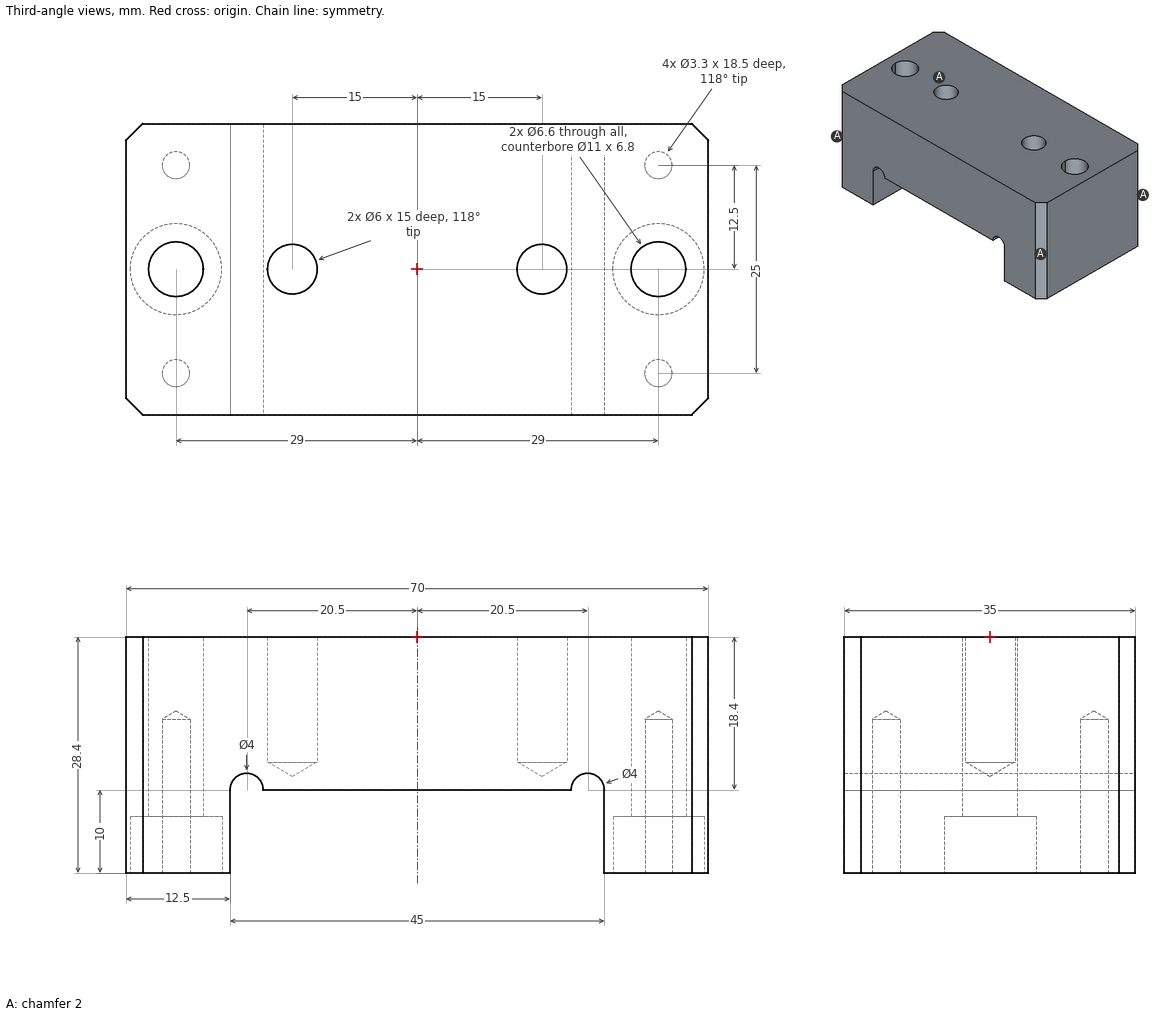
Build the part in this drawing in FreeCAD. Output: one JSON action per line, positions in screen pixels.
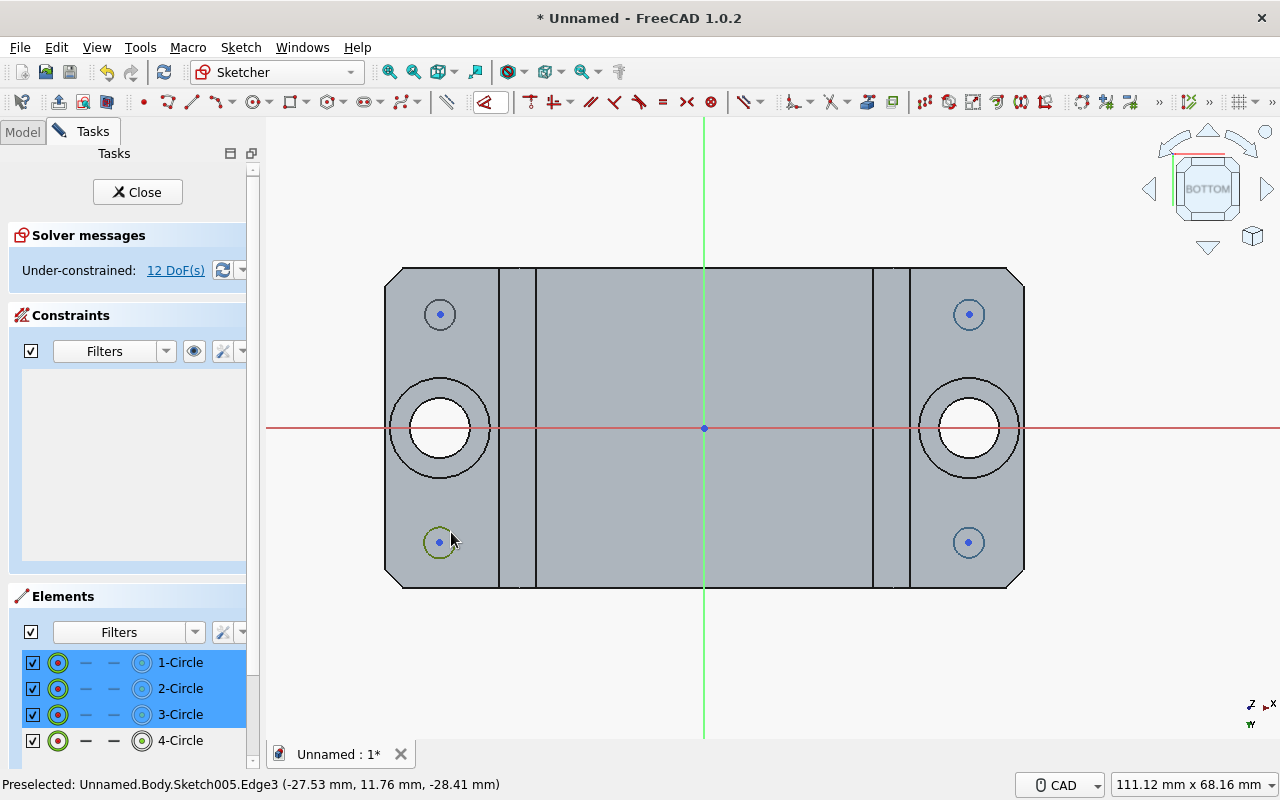
{"action": "left_click", "coordinate": [451, 304]}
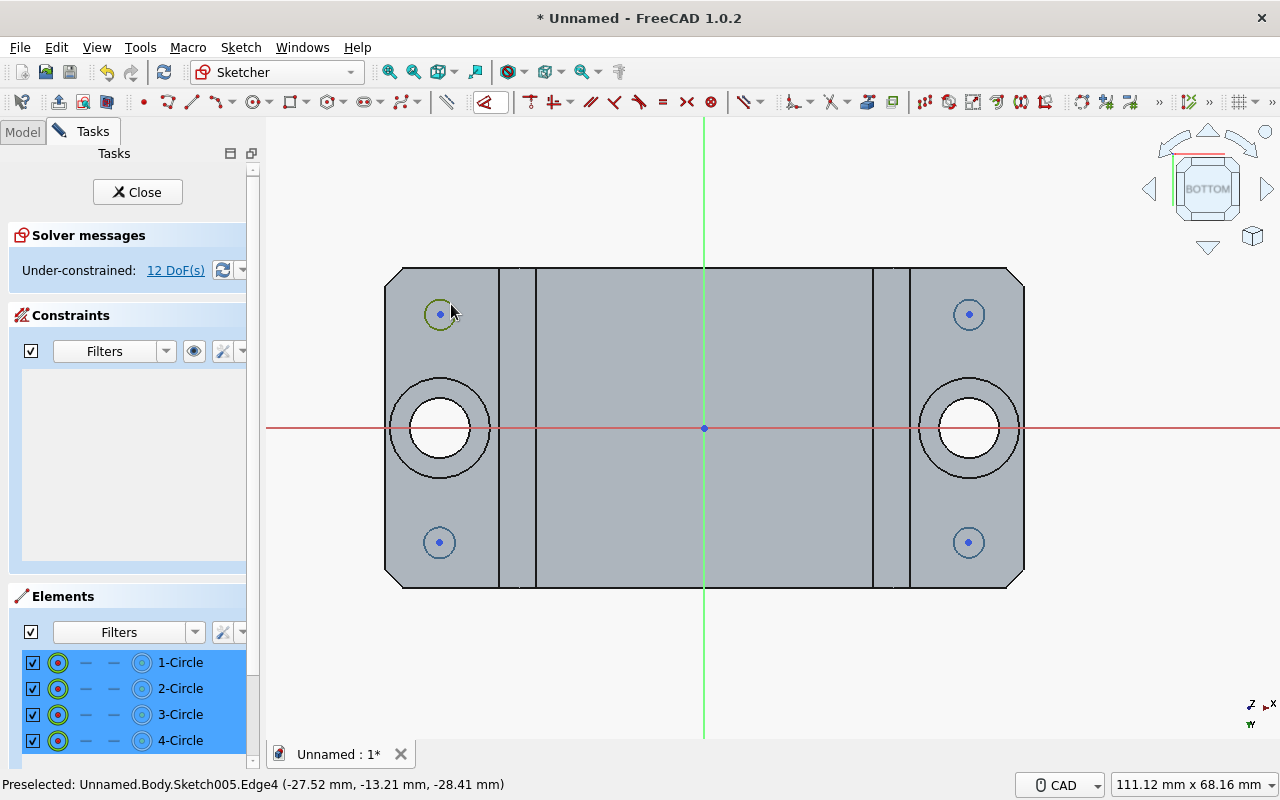
{"action": "key", "text": "e"}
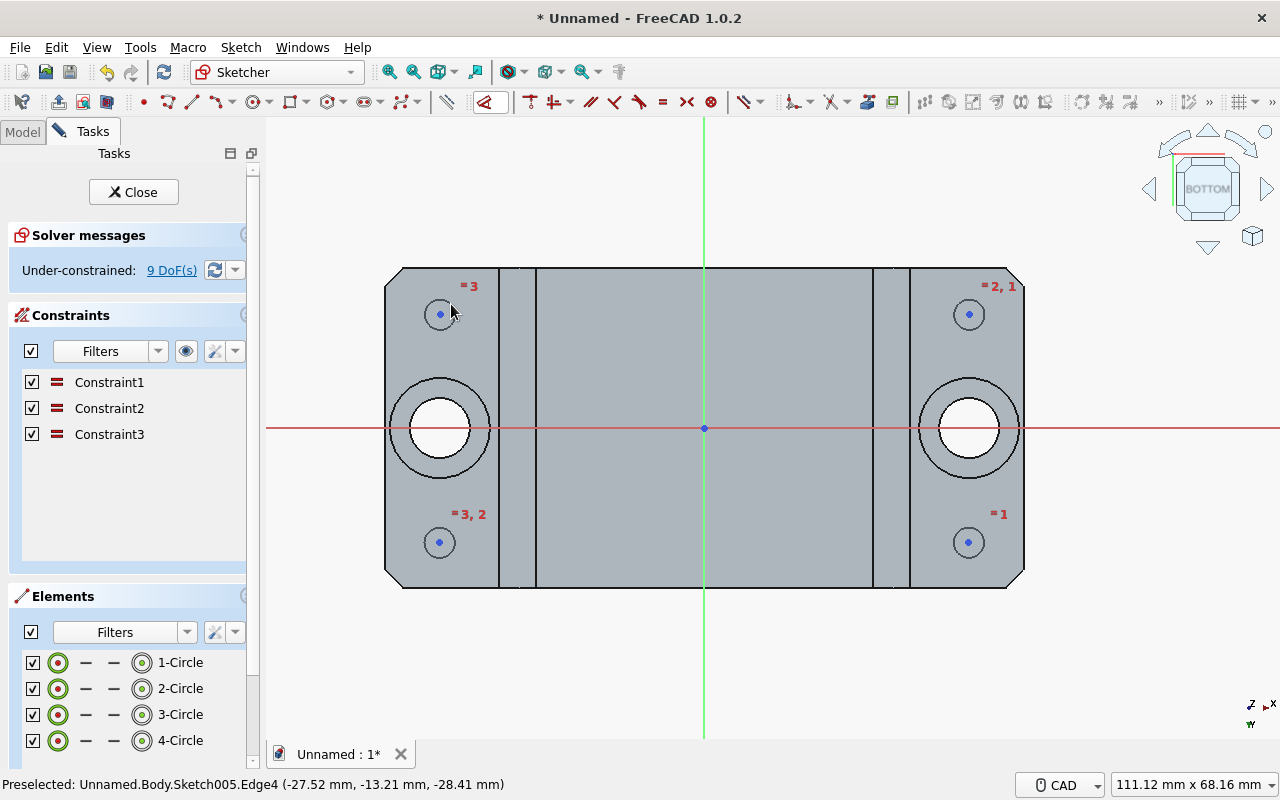
{"action": "left_click", "coordinate": [969, 543]}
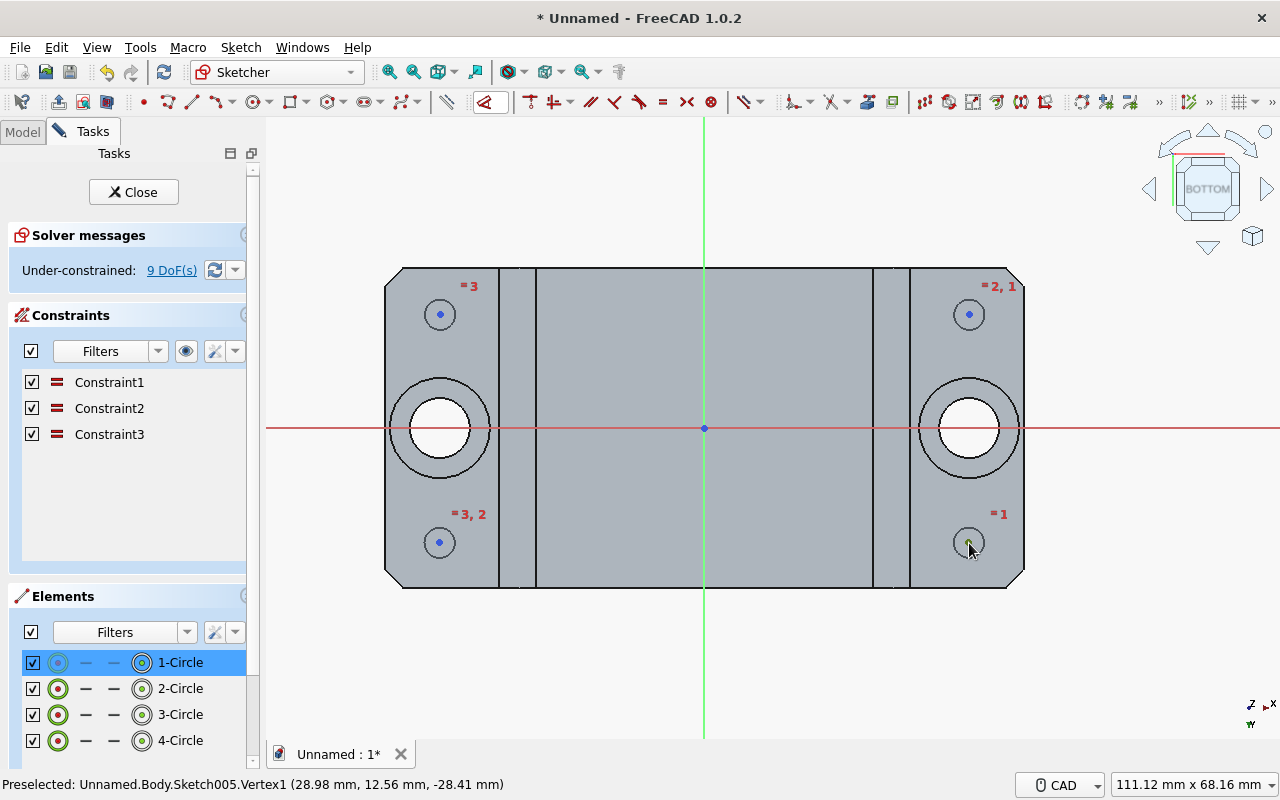
{"action": "left_click", "coordinate": [969, 315]}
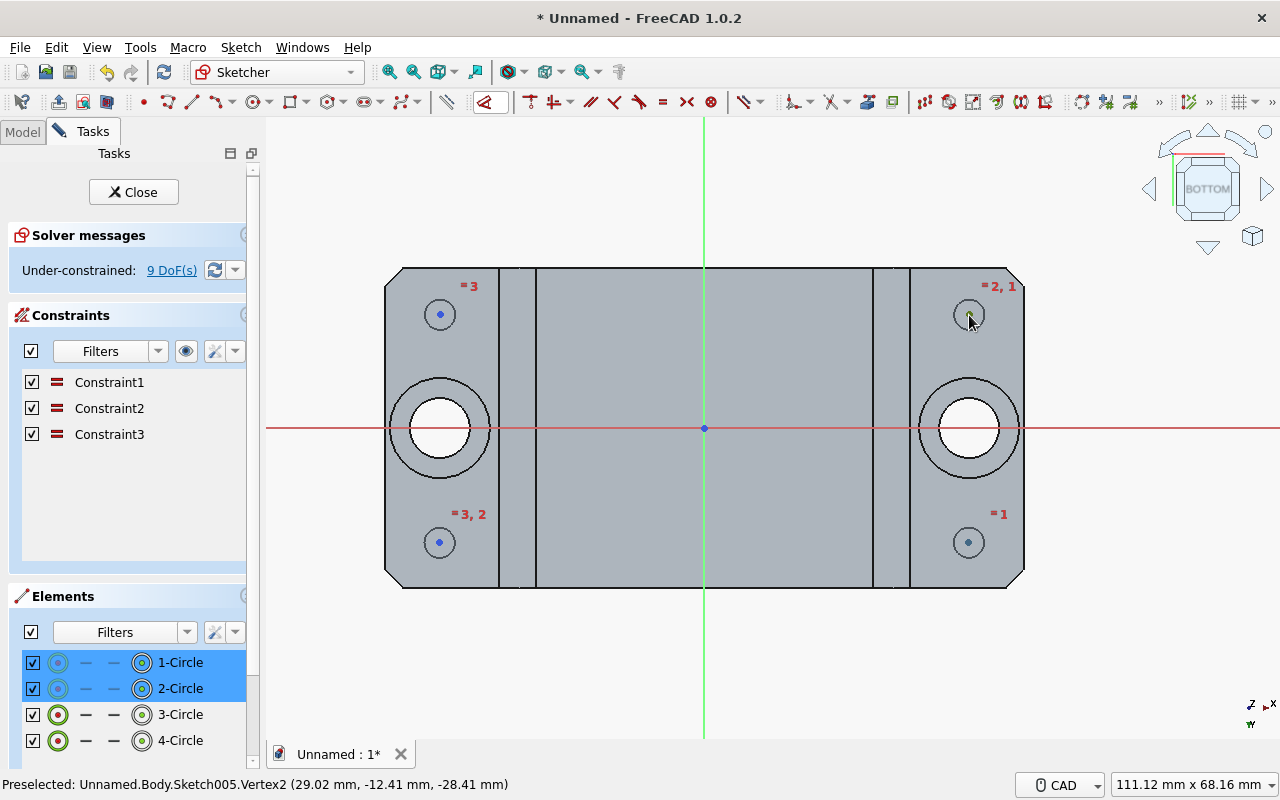
{"action": "key", "text": "v"}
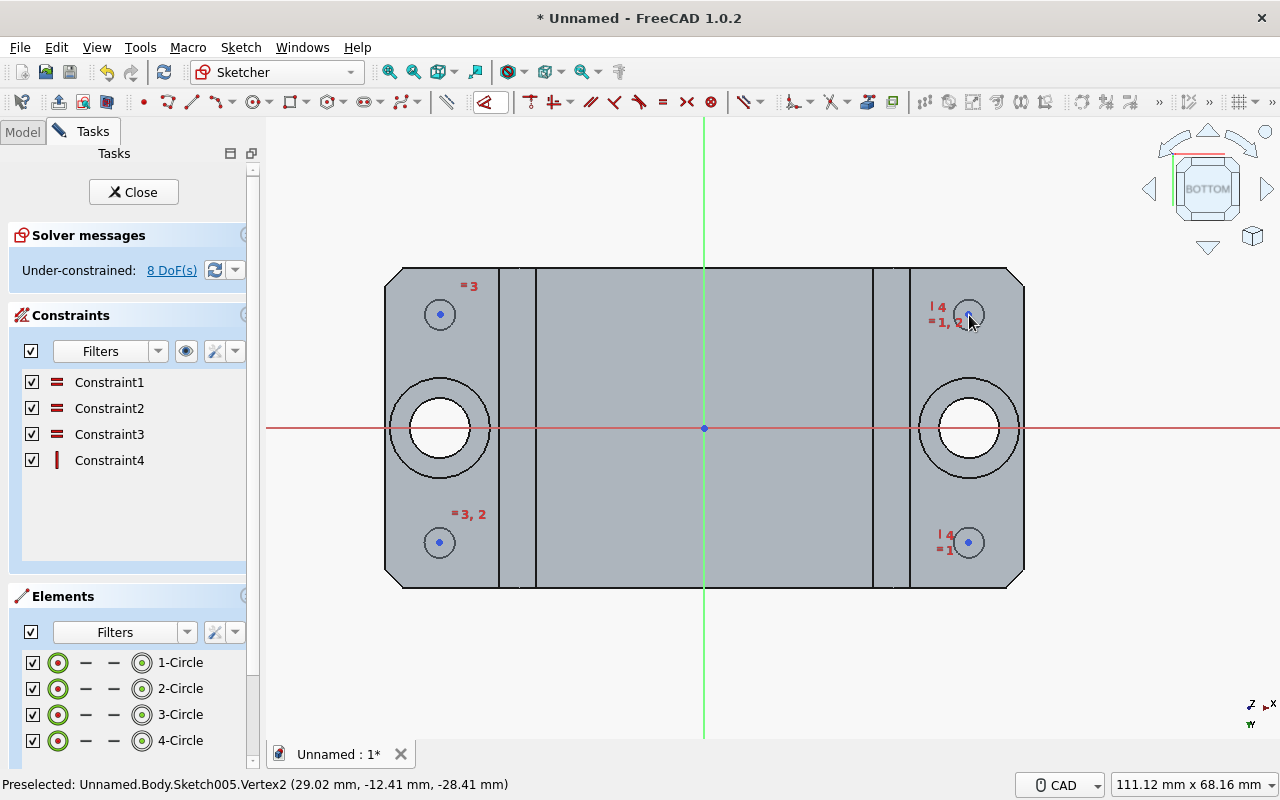
{"action": "left_click", "coordinate": [969, 543]}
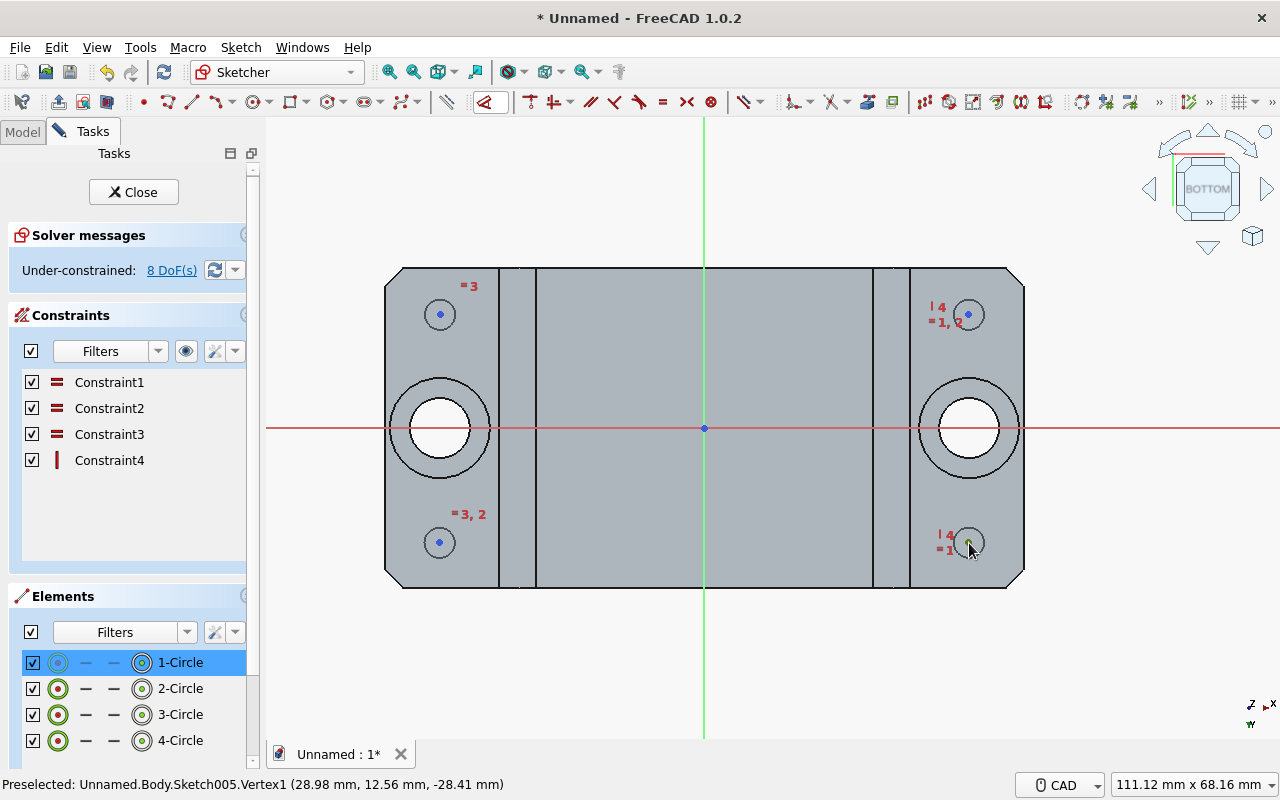
{"action": "left_click", "coordinate": [440, 543]}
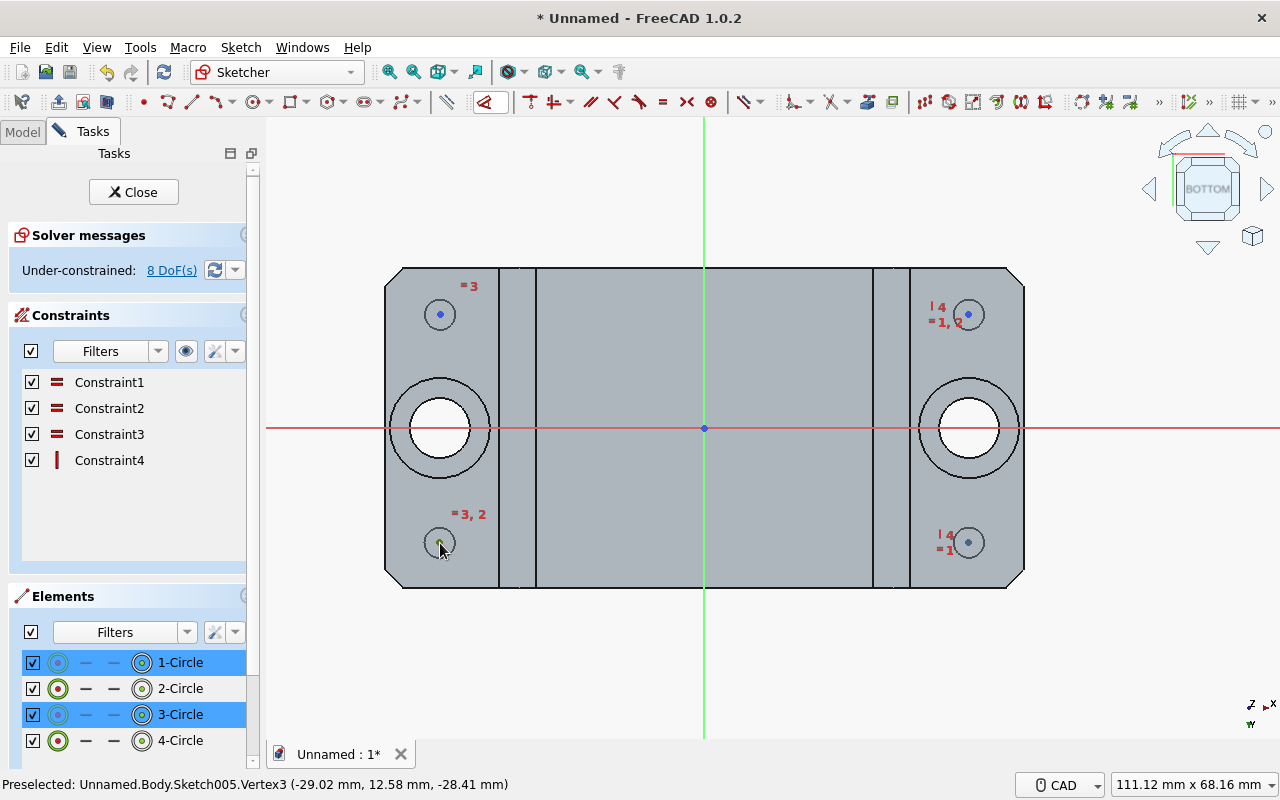
{"action": "key", "text": "h"}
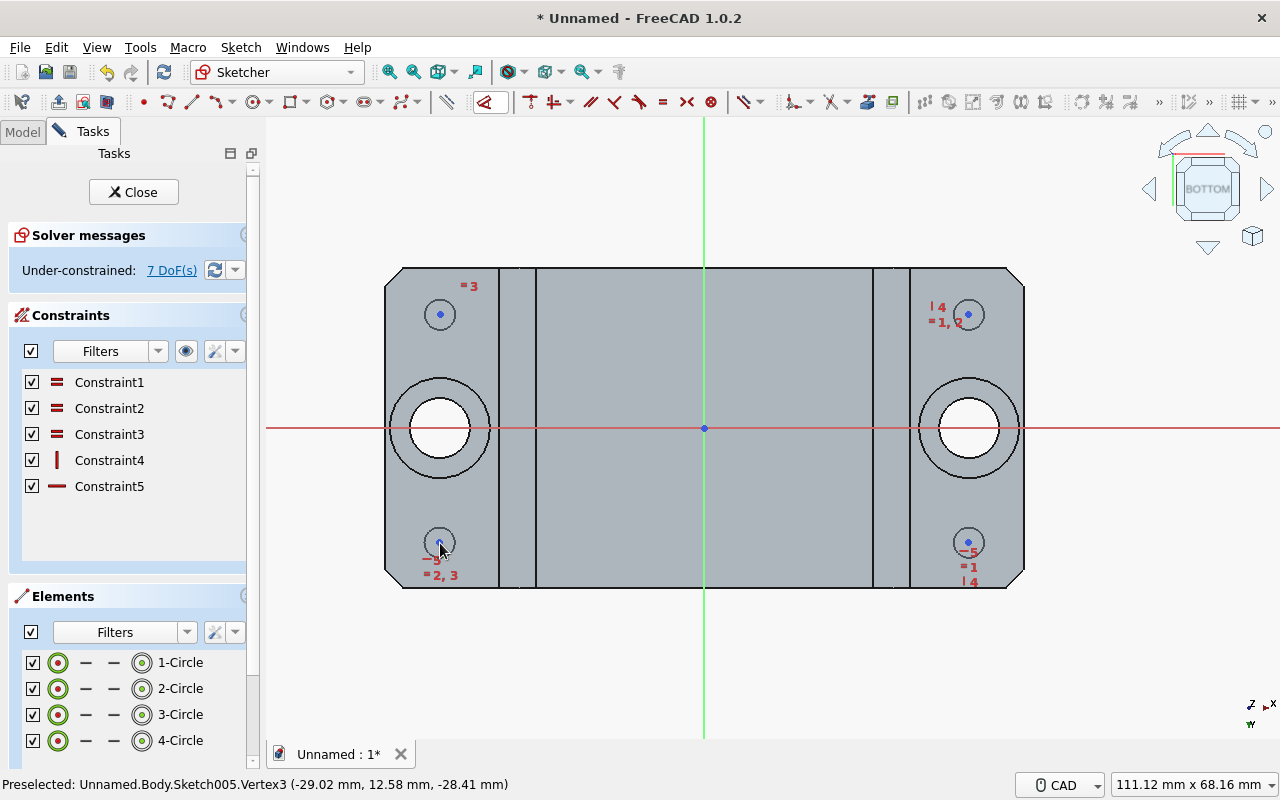
{"action": "left_click", "coordinate": [440, 543]}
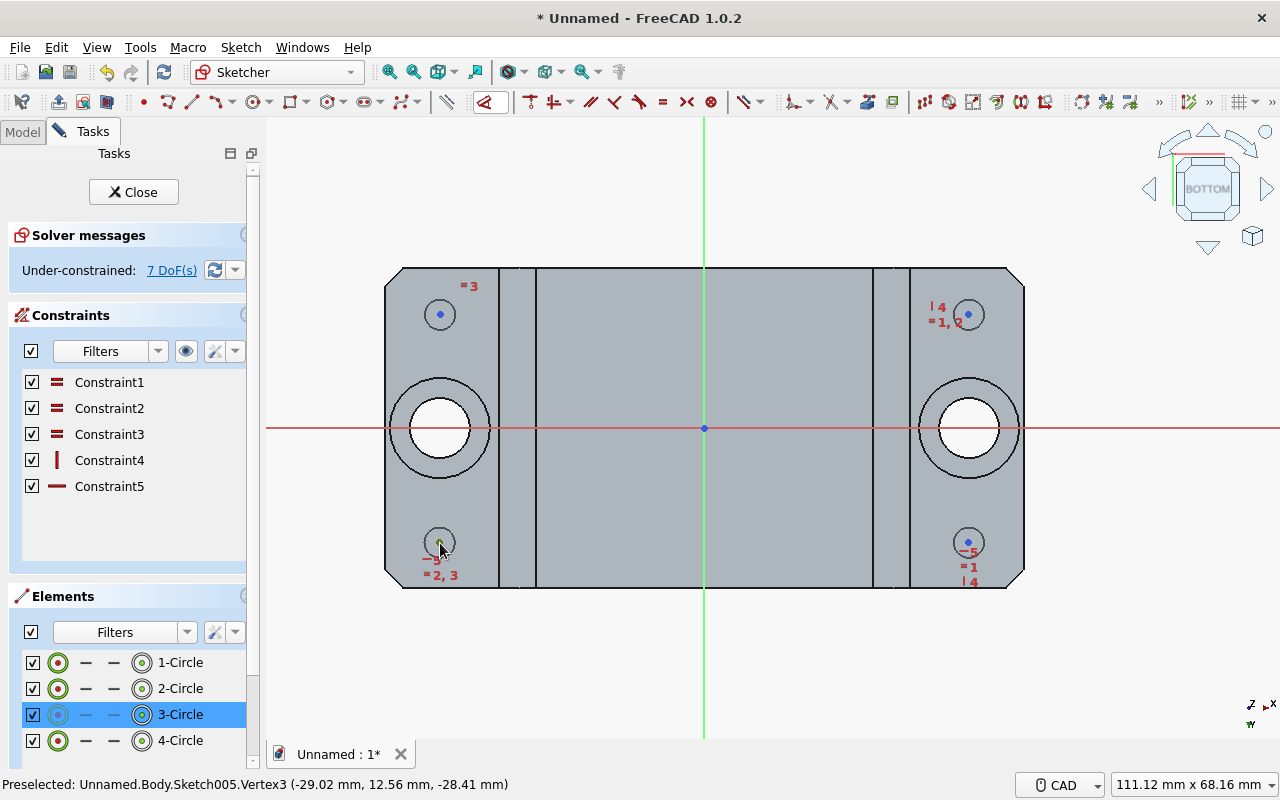
{"action": "left_click", "coordinate": [440, 315]}